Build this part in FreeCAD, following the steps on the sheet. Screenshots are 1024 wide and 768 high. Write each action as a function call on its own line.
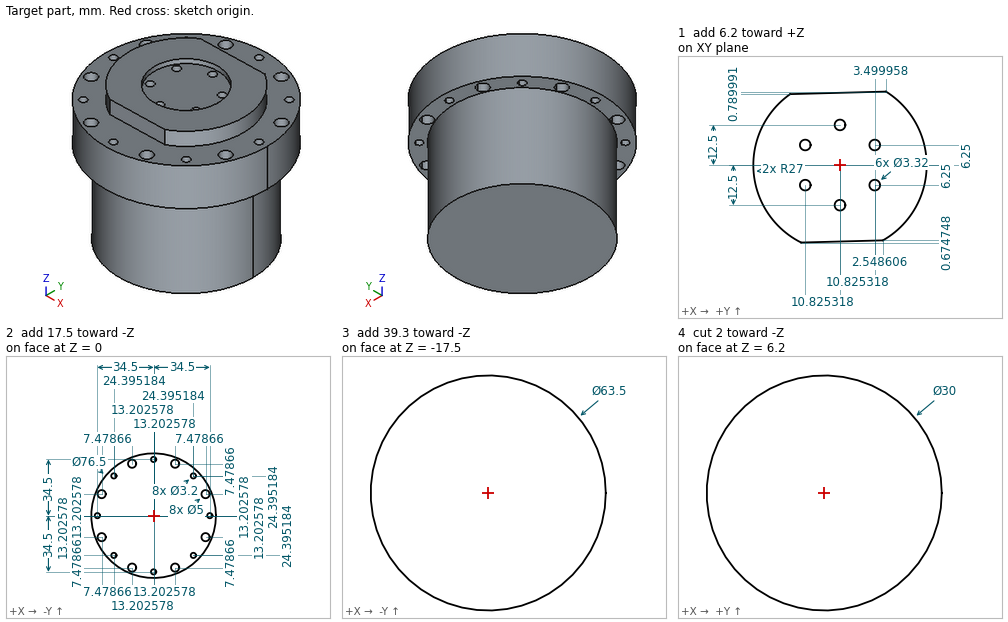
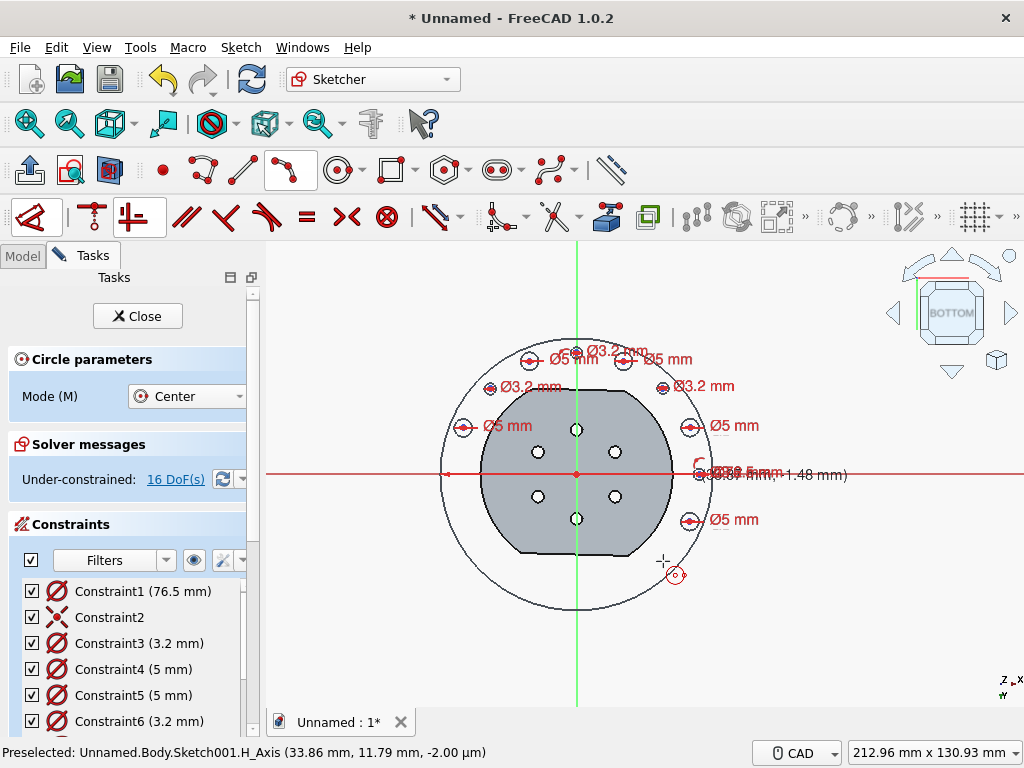
click(663, 561)
move(659, 557)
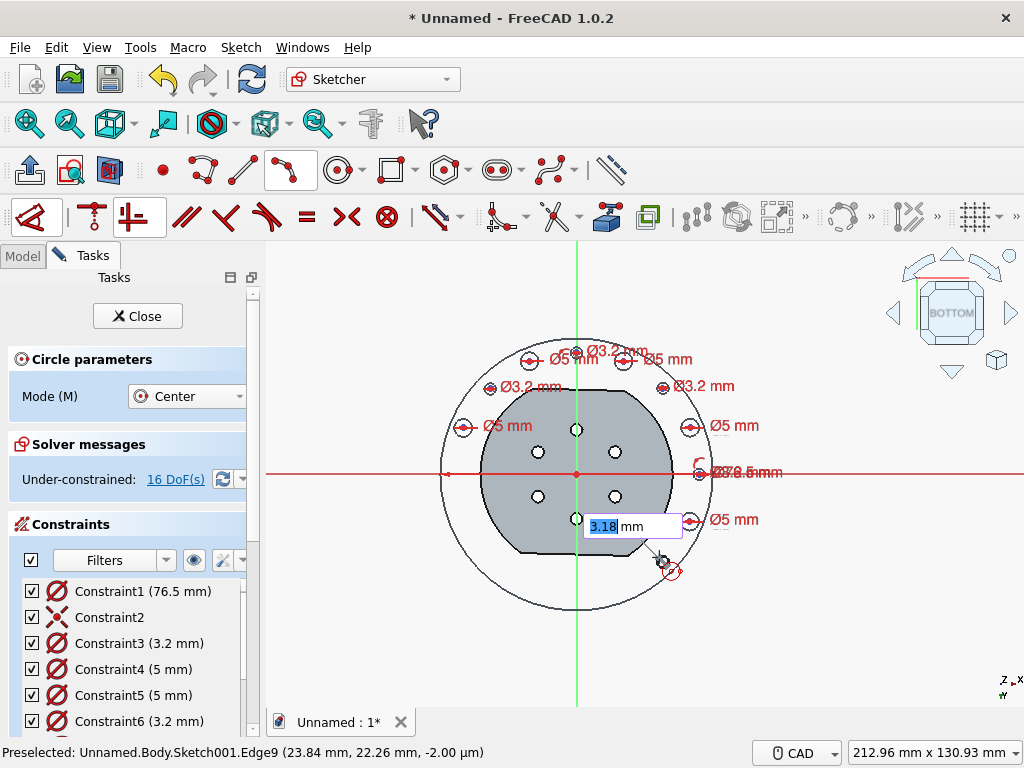
text(3.2)
key(Return)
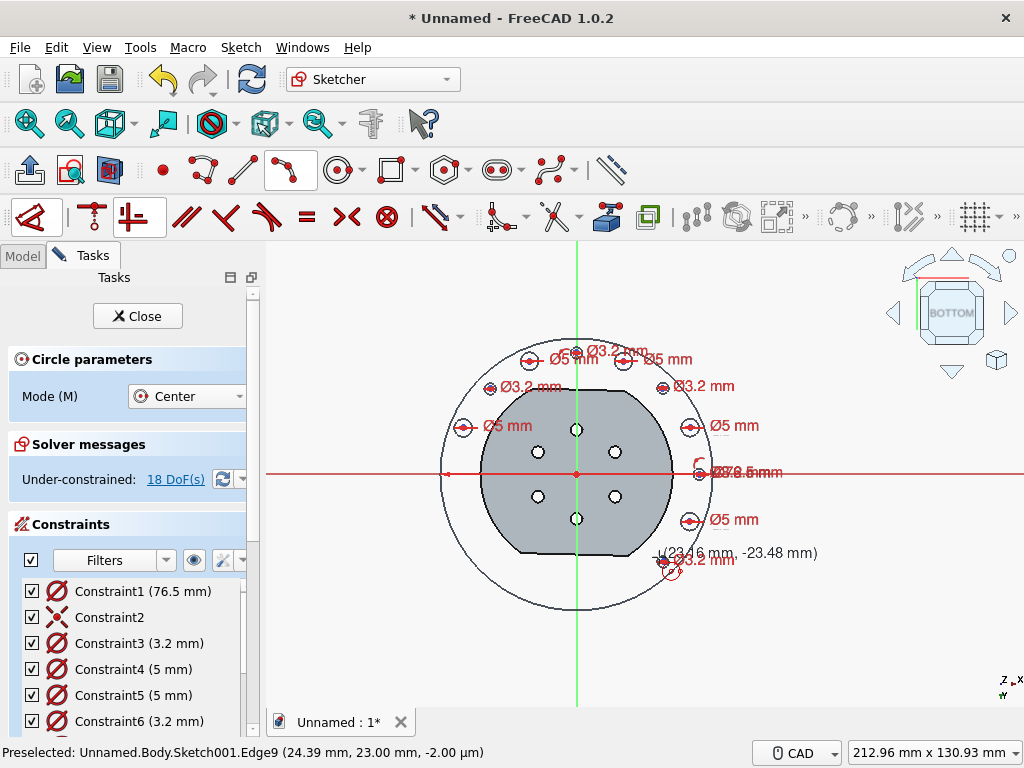
scroll(624, 588, up, 5)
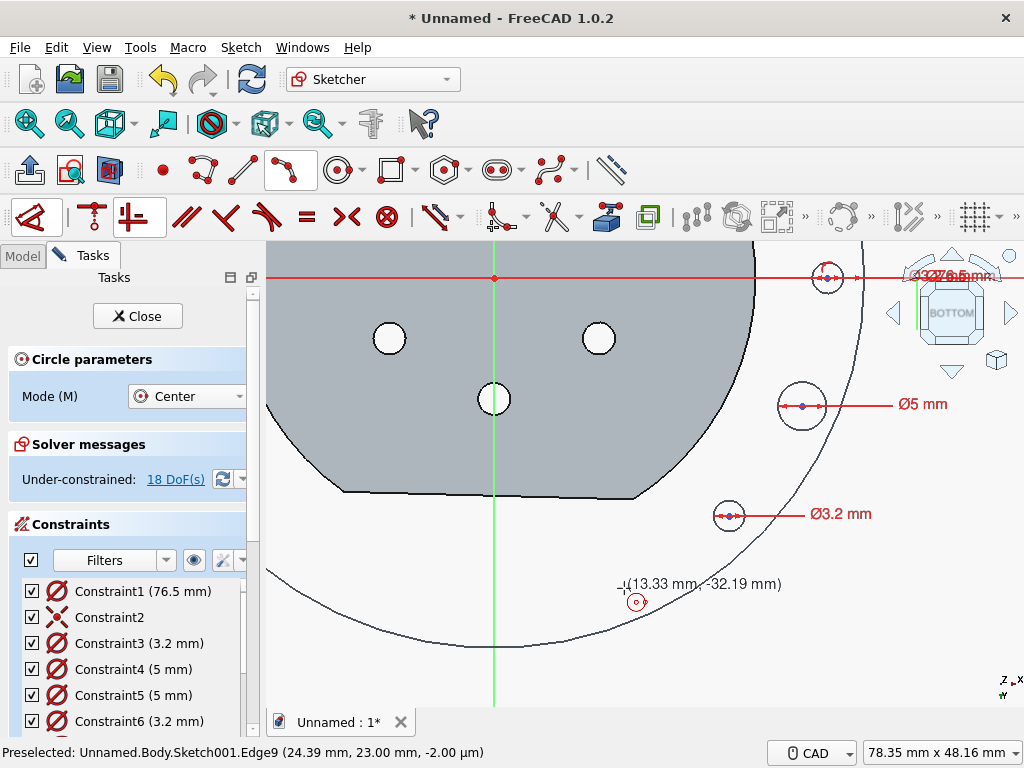
click(622, 586)
move(639, 569)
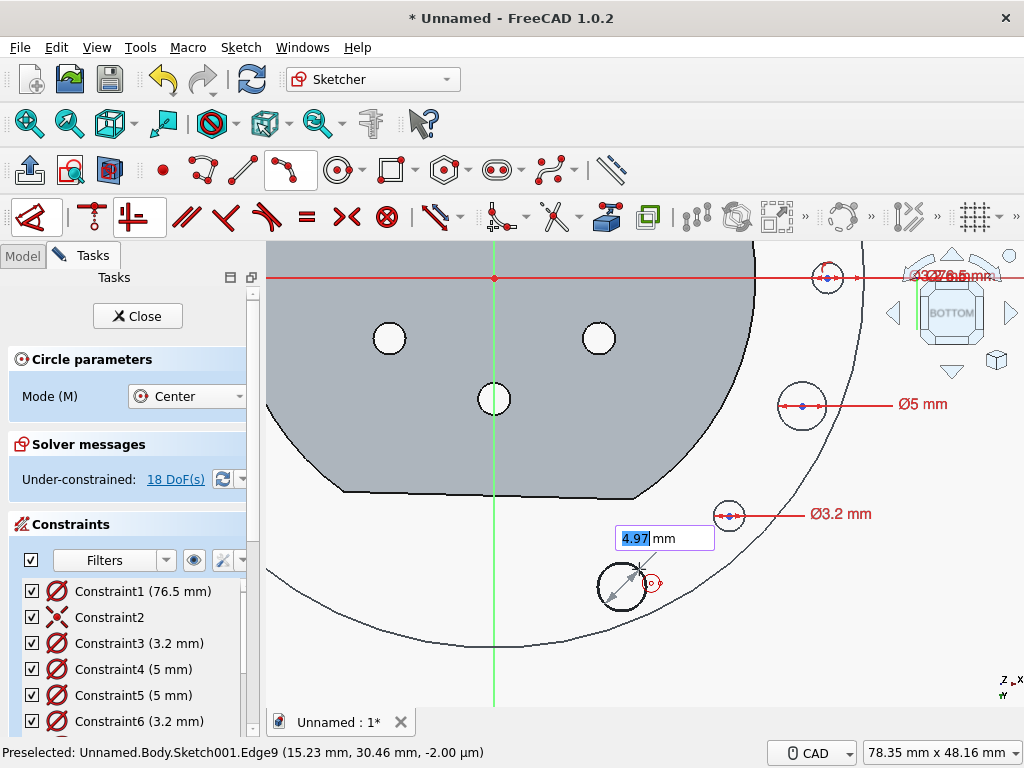
text(5)
key(Return)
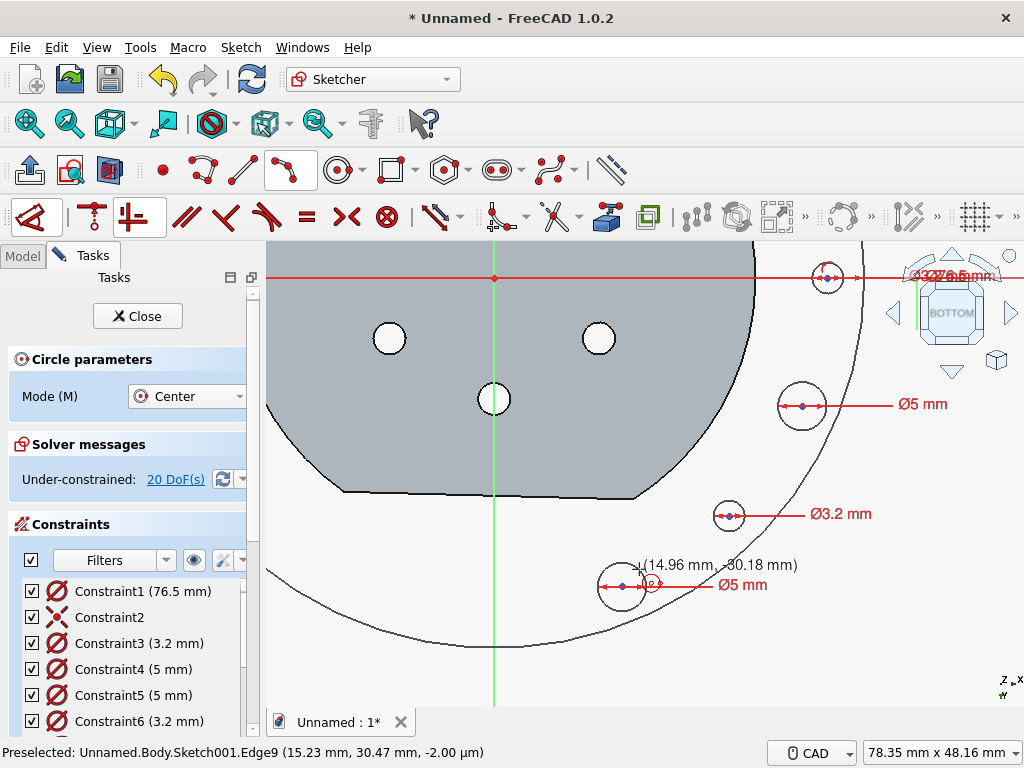
scroll(624, 588, down, 5)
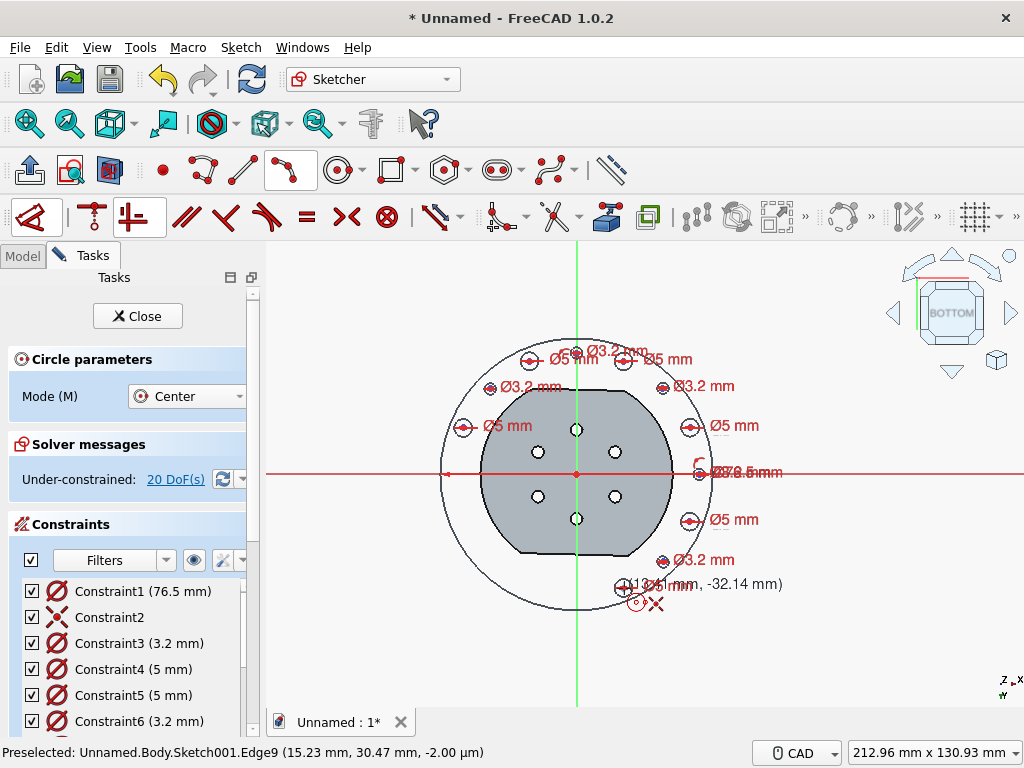
scroll(454, 474, up, 7)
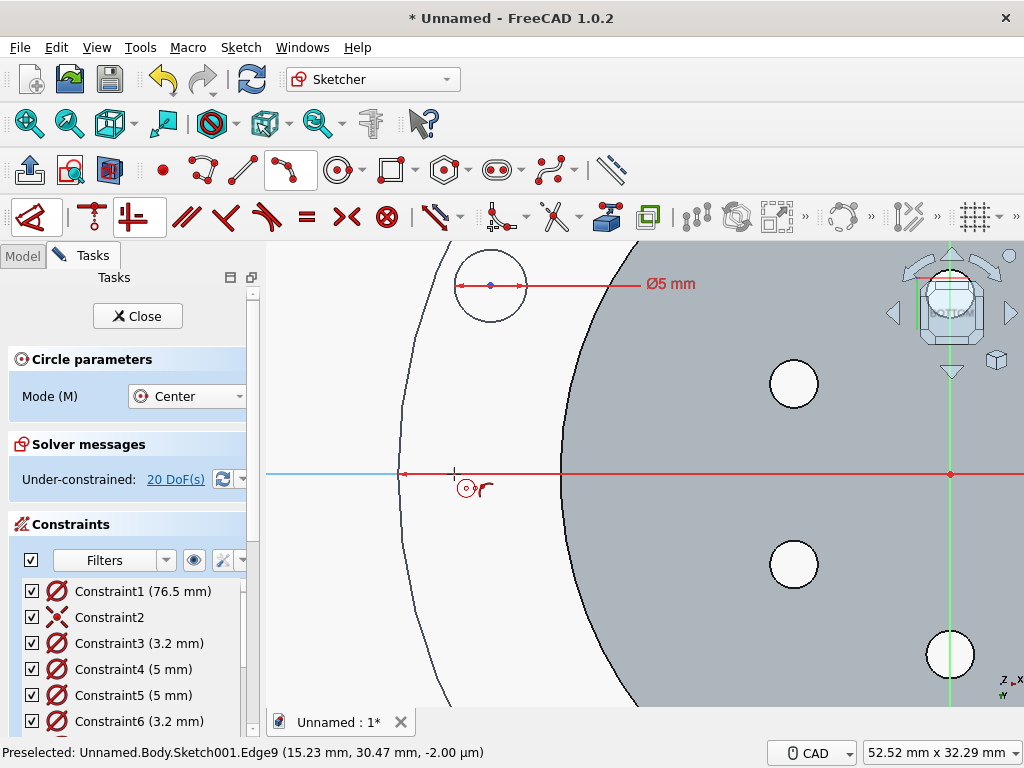
scroll(454, 474, down, 7)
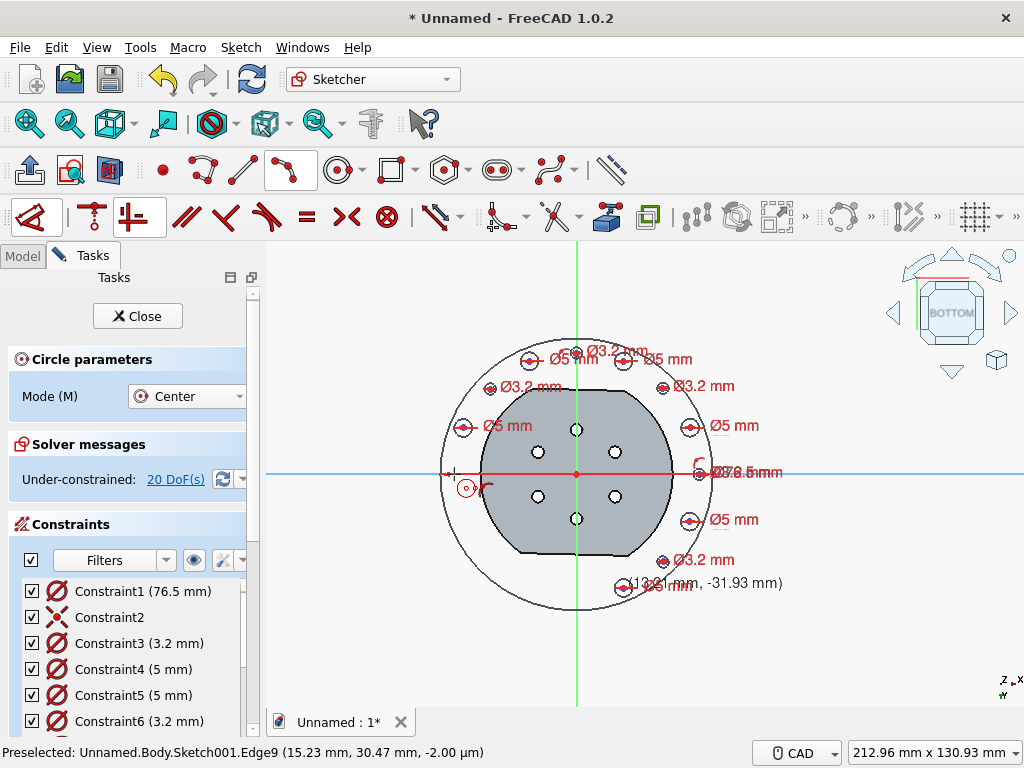
click(454, 474)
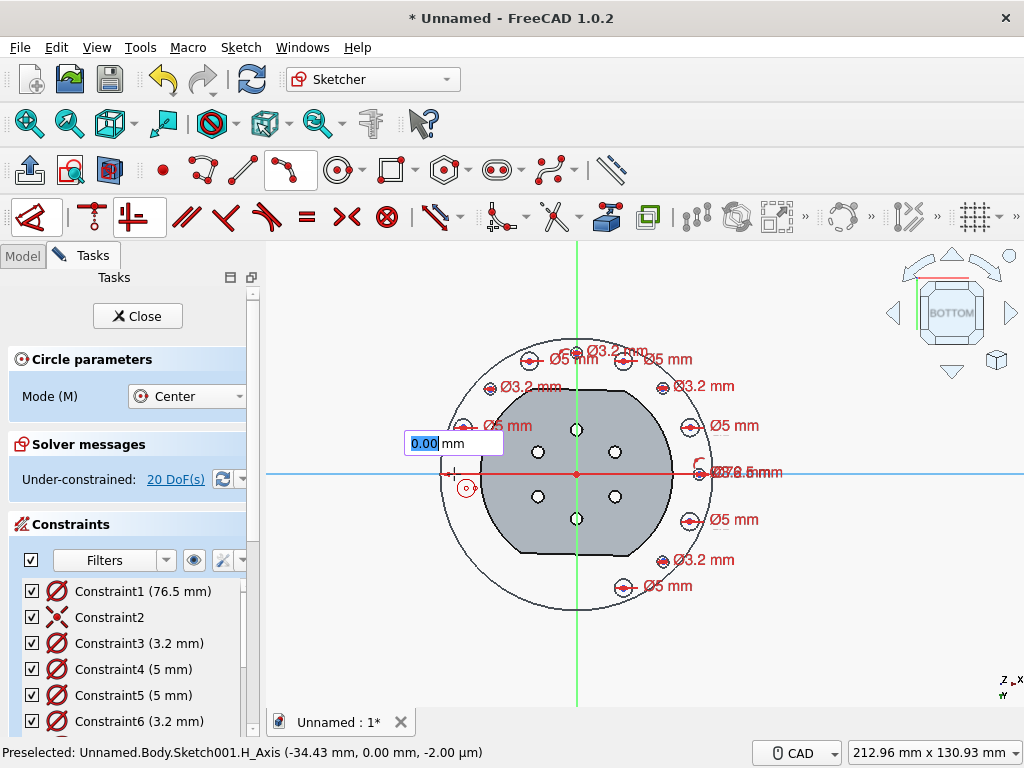
scroll(452, 480, up, 6)
move(451, 478)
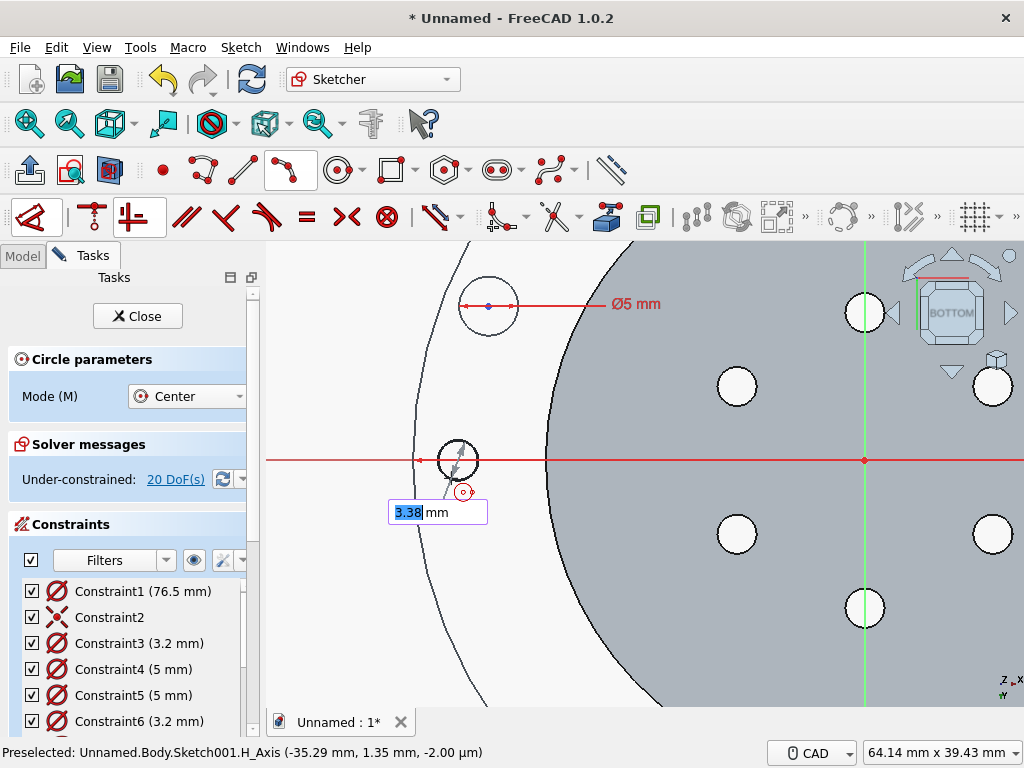
text(3.2)
key(Return)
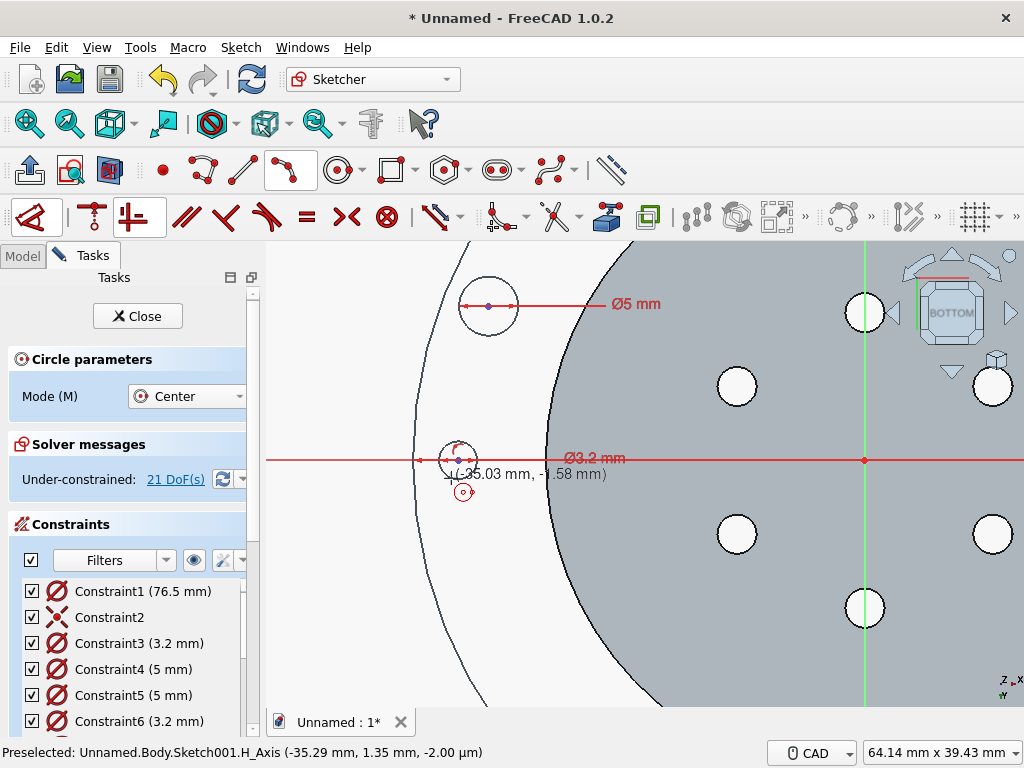
click(488, 616)
move(509, 595)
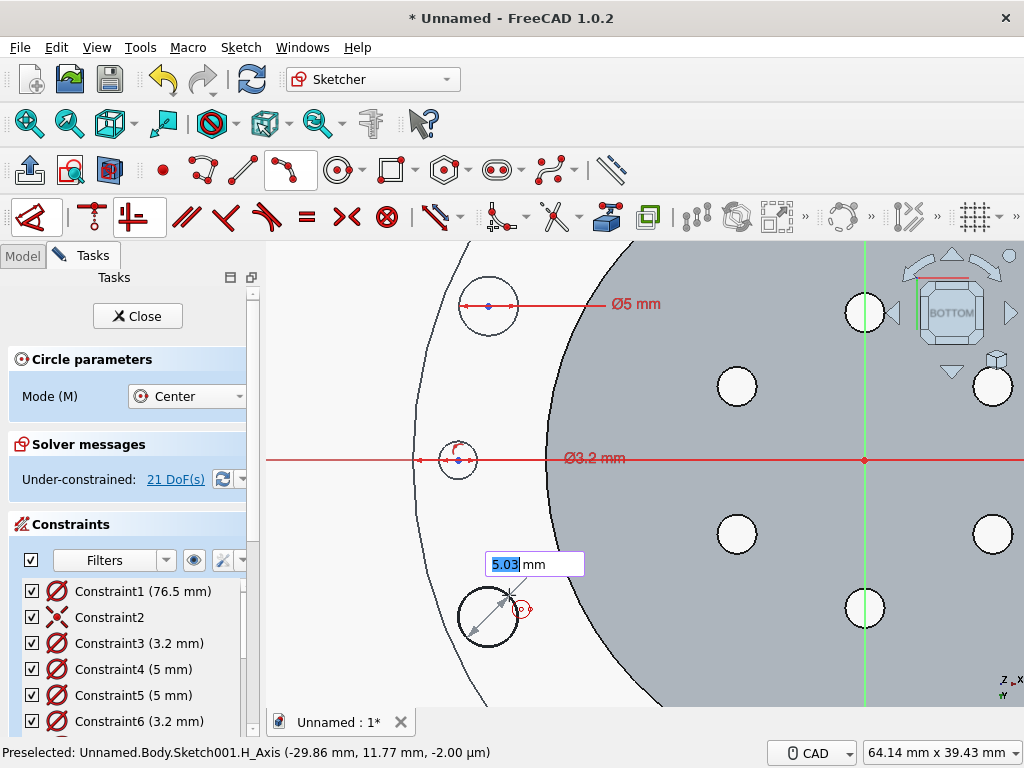
text(5)
key(Return)